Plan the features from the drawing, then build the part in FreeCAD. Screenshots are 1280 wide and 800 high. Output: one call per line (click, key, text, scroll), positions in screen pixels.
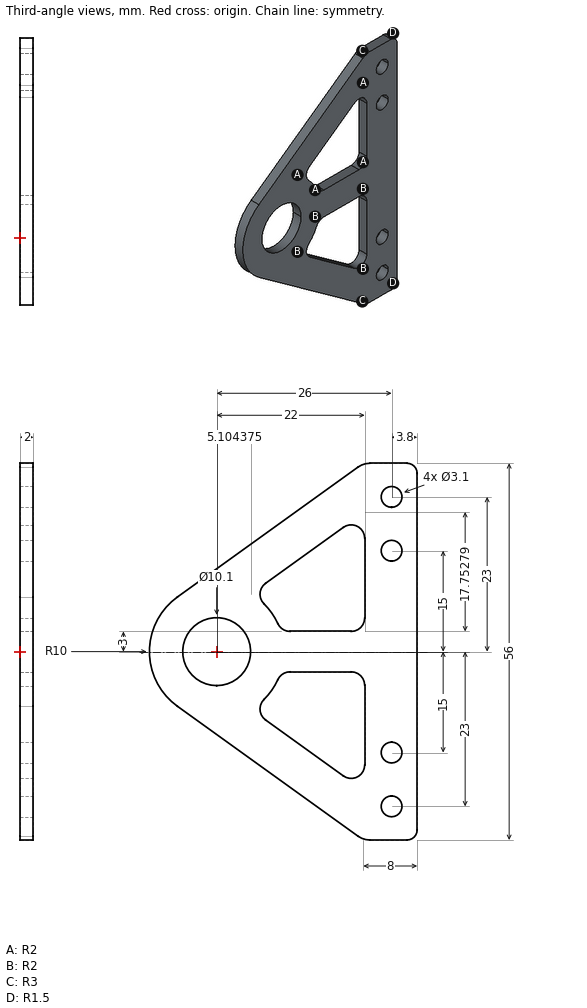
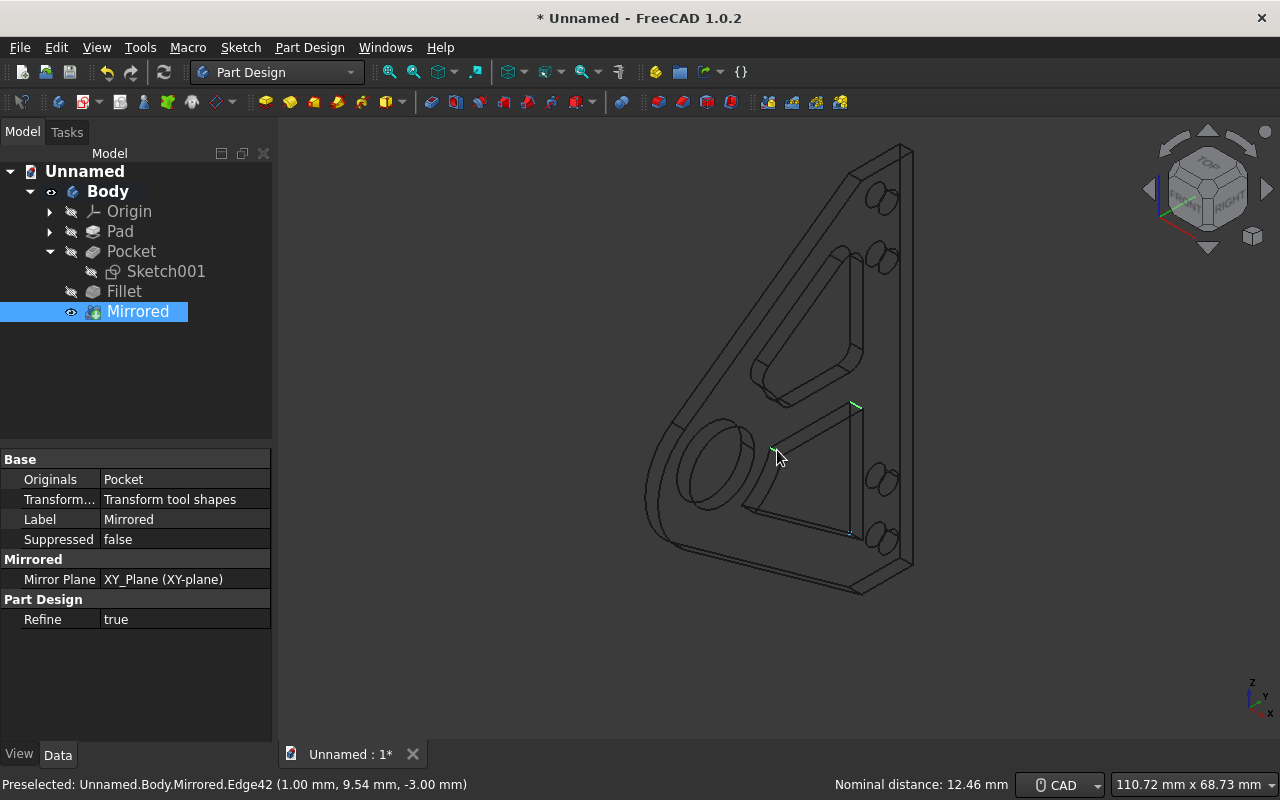
click(748, 508, ctrl)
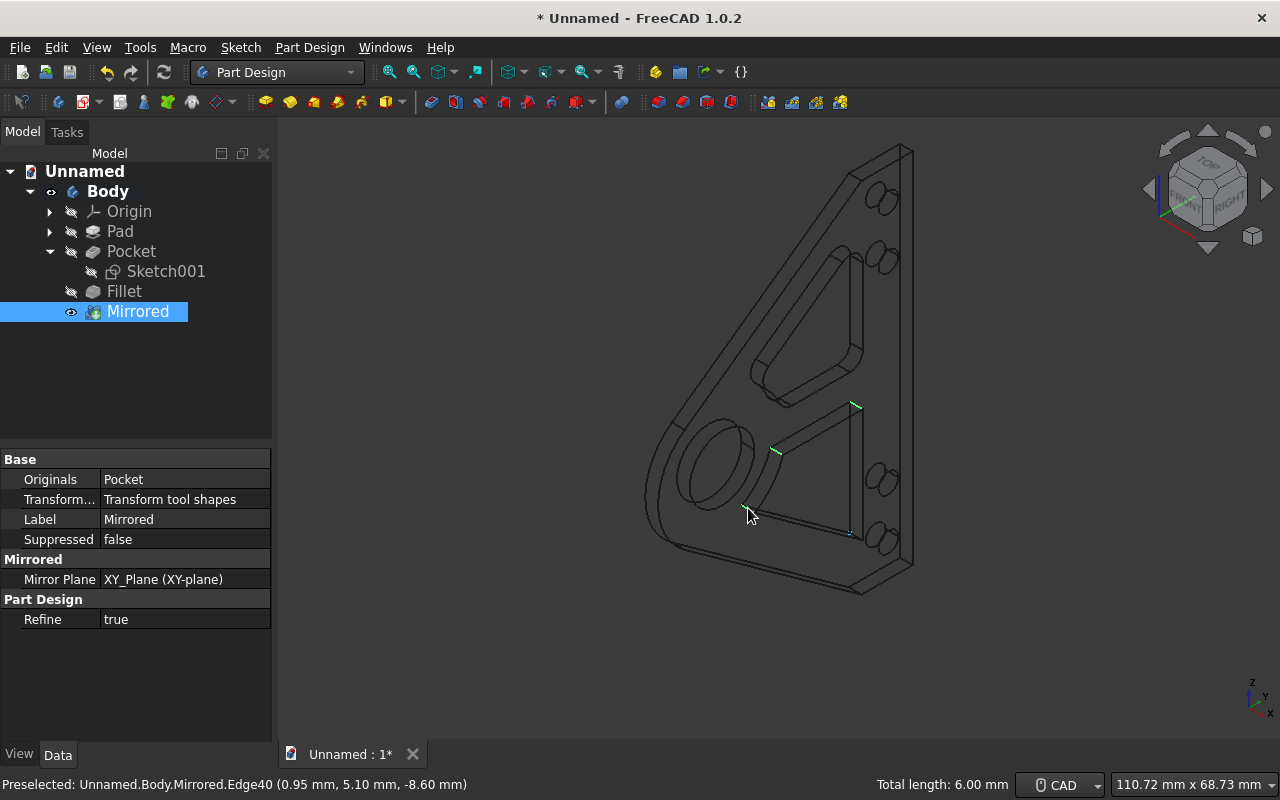
scroll(856, 536, up, 4)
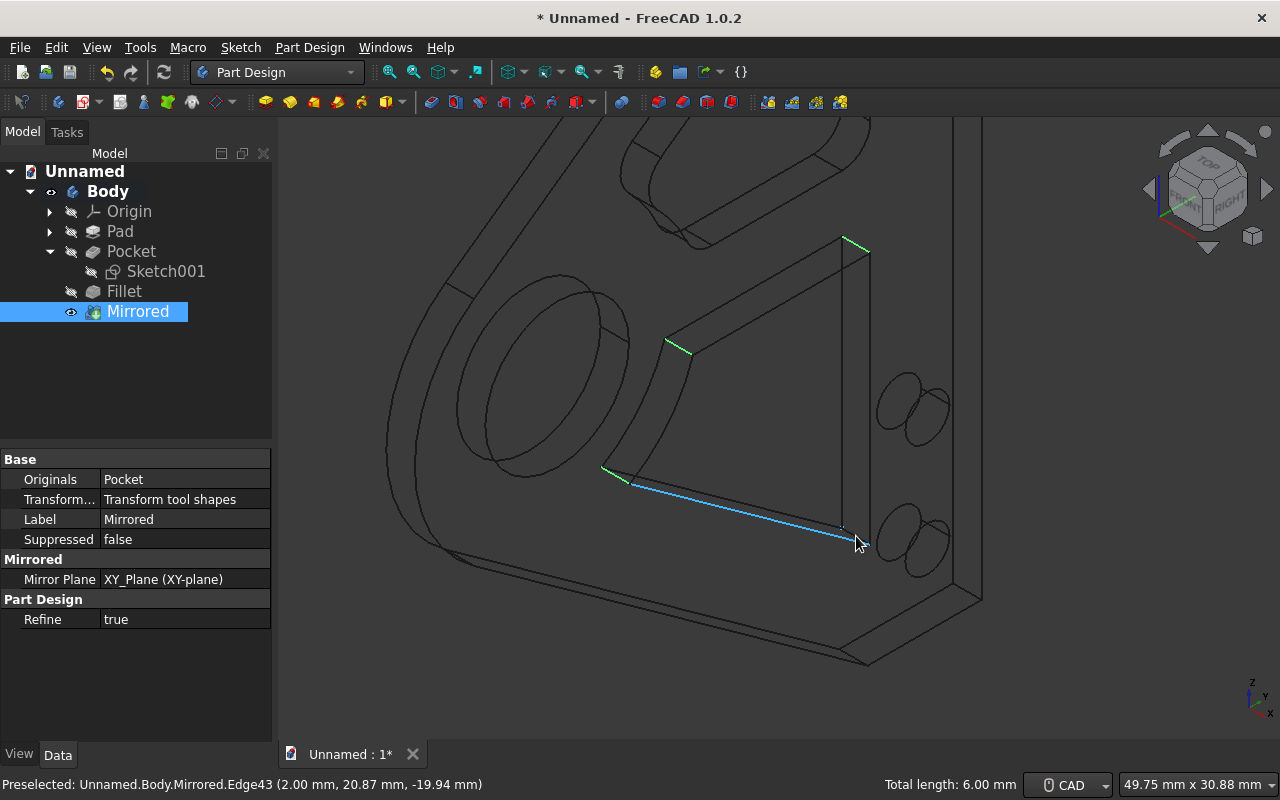
click(851, 532, ctrl)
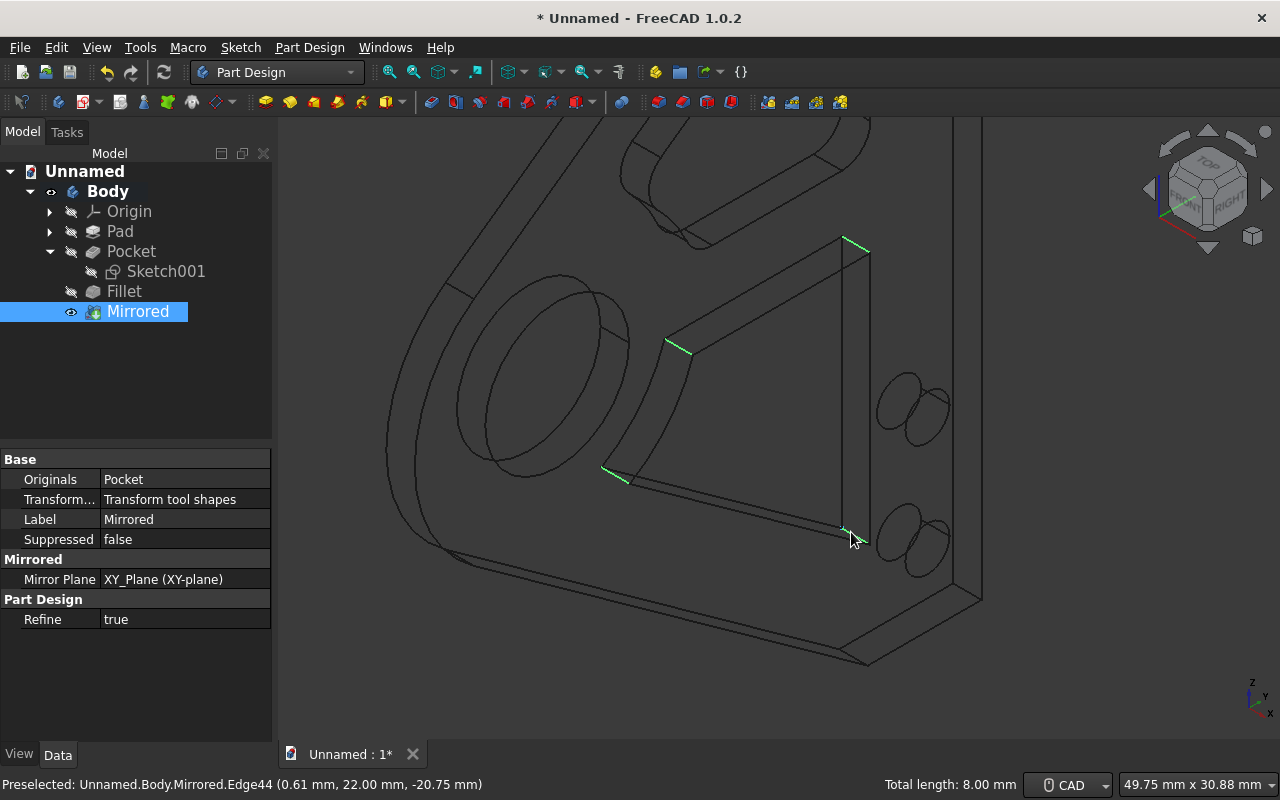
key(v)
key(1)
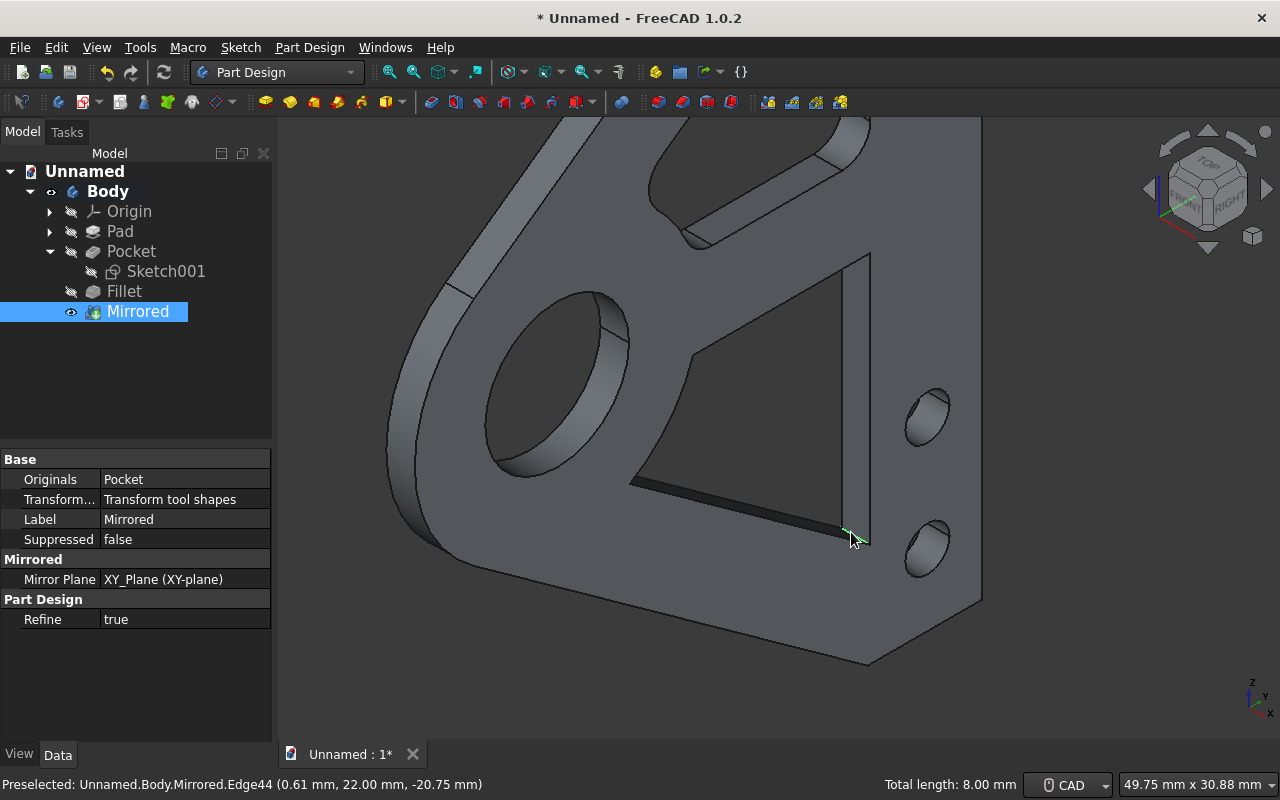
click(660, 102)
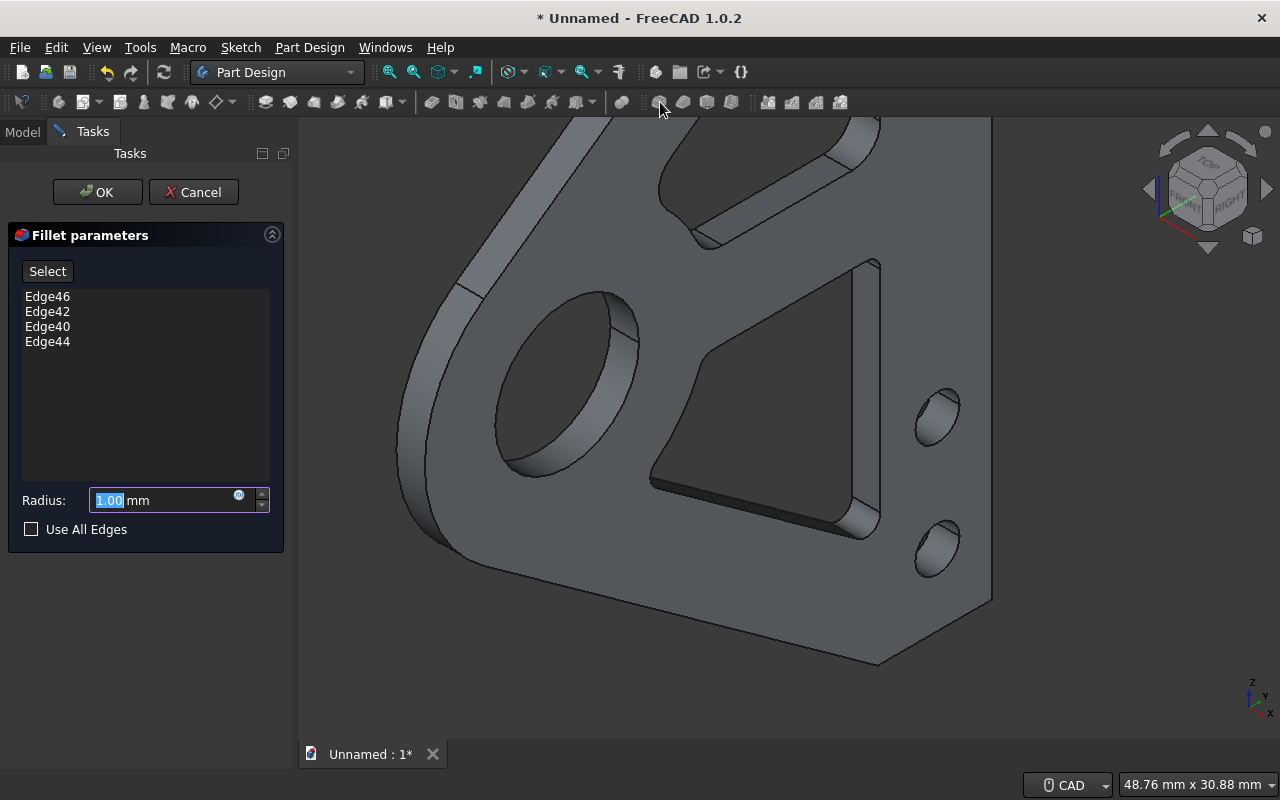
text(2)
key(Tab)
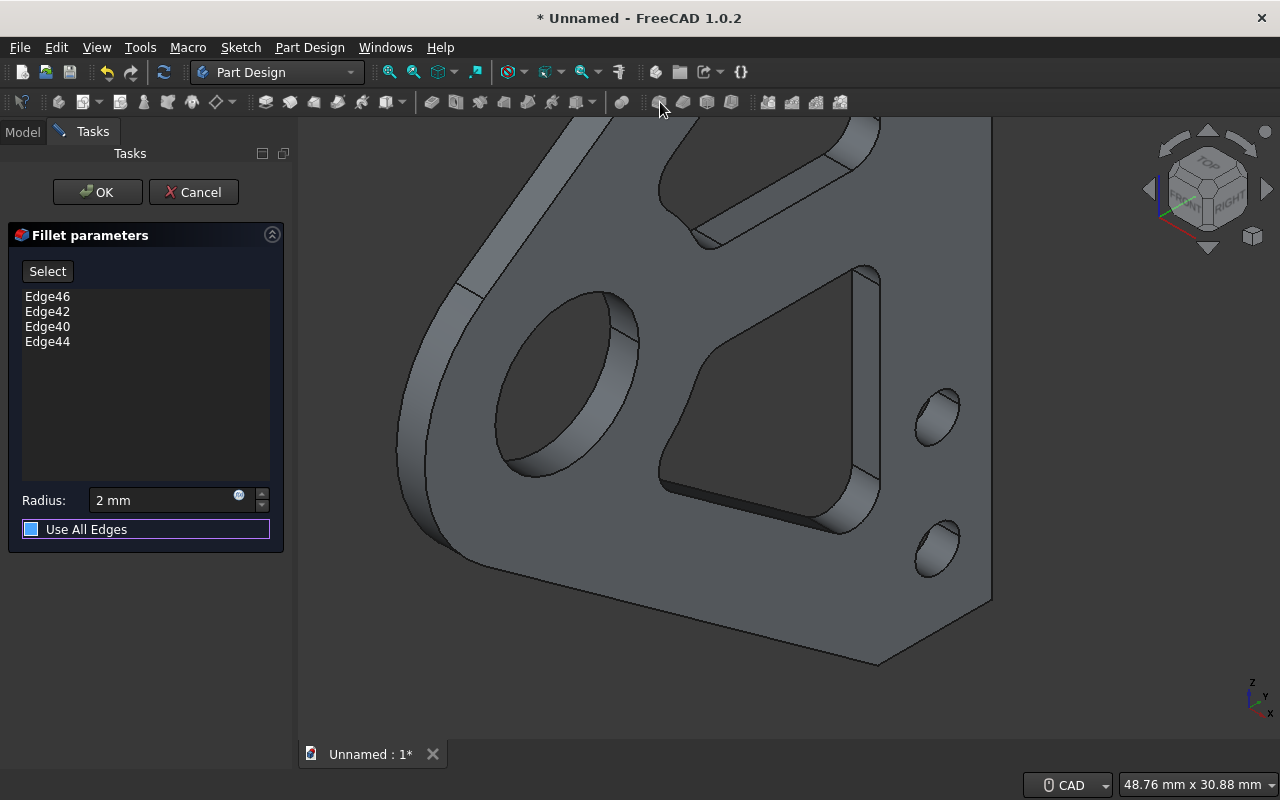
click(98, 192)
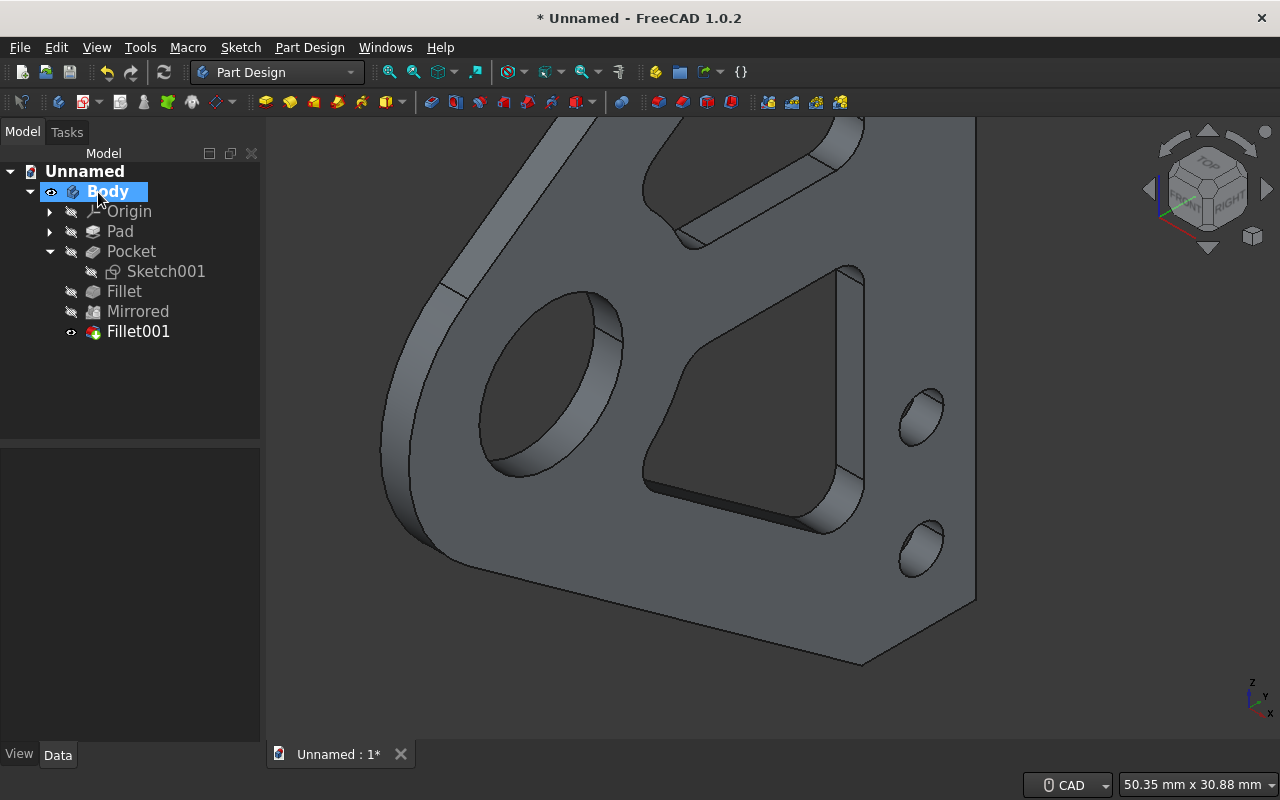
click(390, 72)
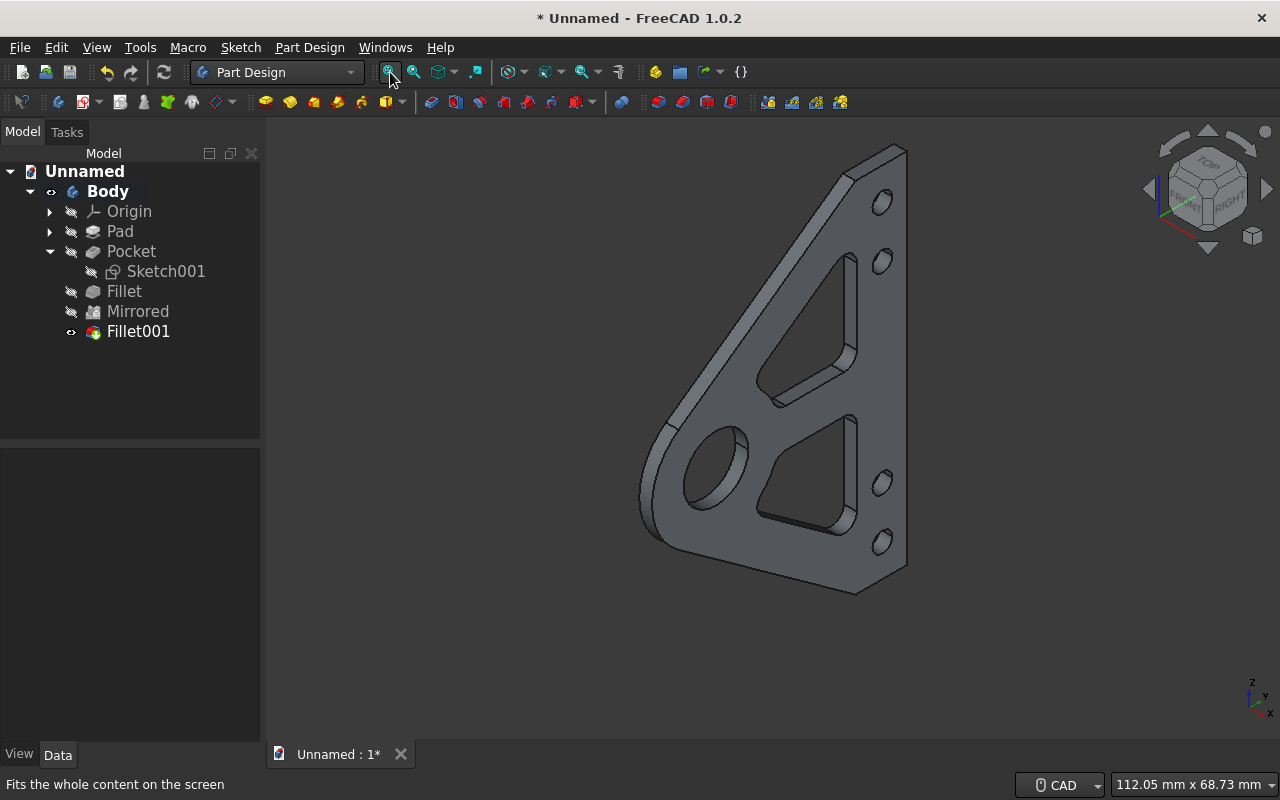
scroll(849, 590, up, 4)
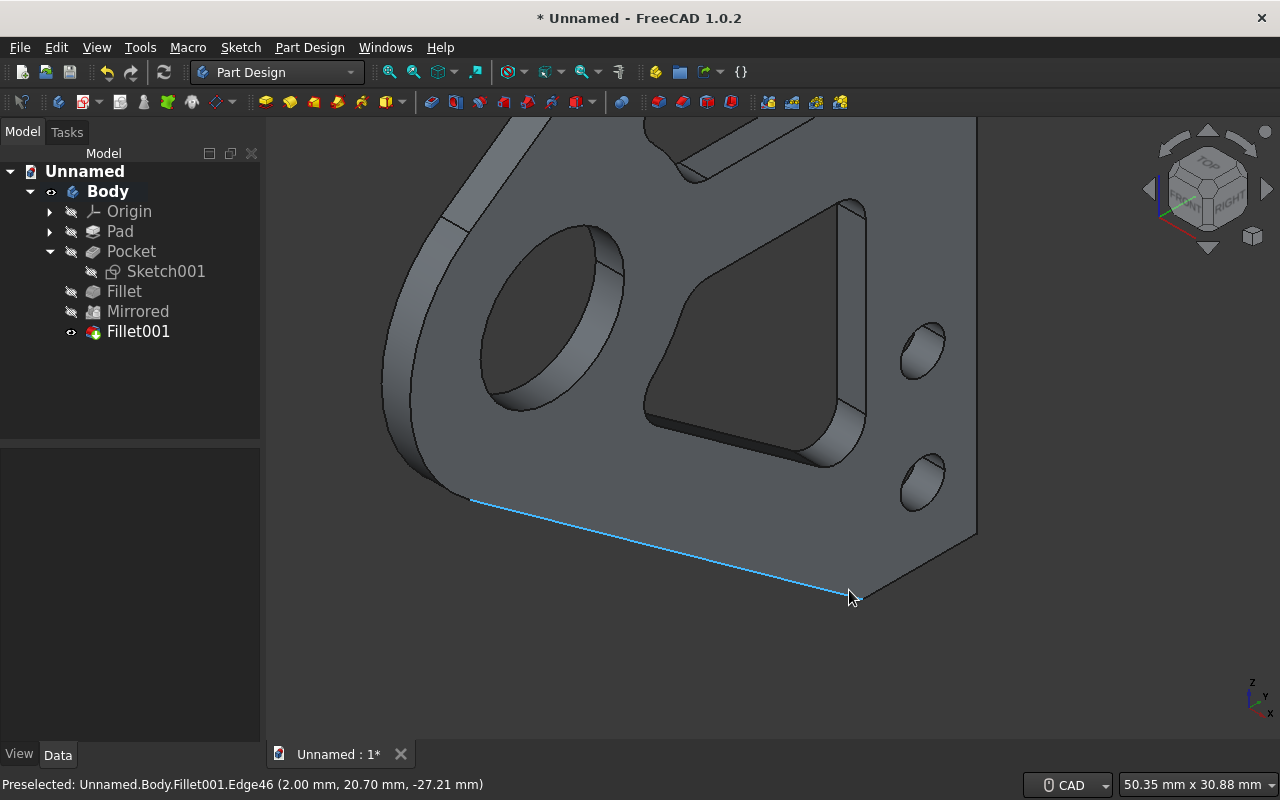
click(390, 72)